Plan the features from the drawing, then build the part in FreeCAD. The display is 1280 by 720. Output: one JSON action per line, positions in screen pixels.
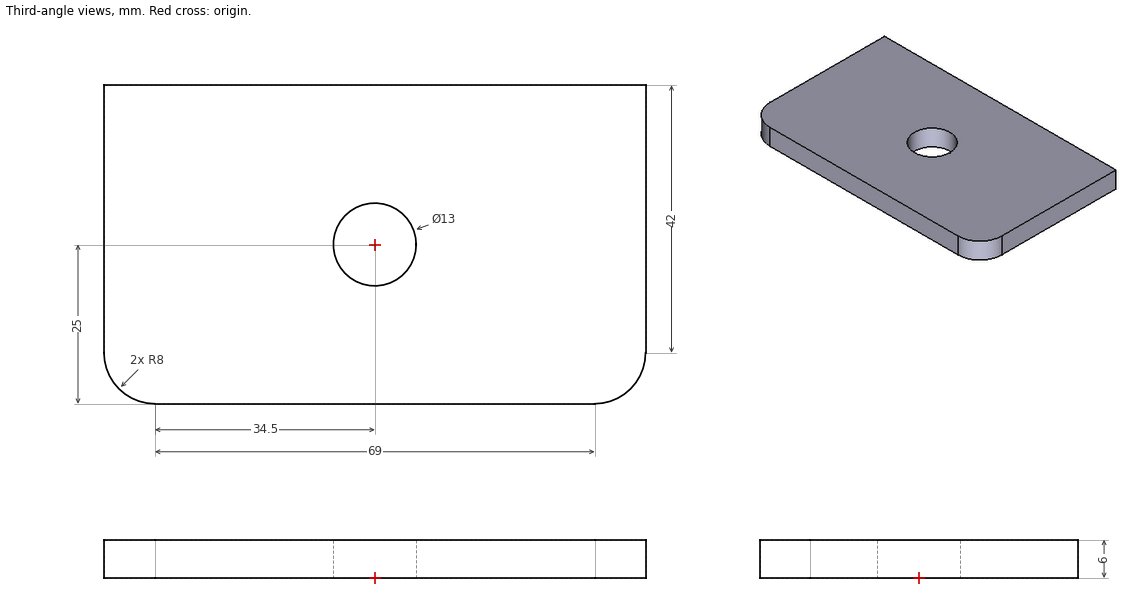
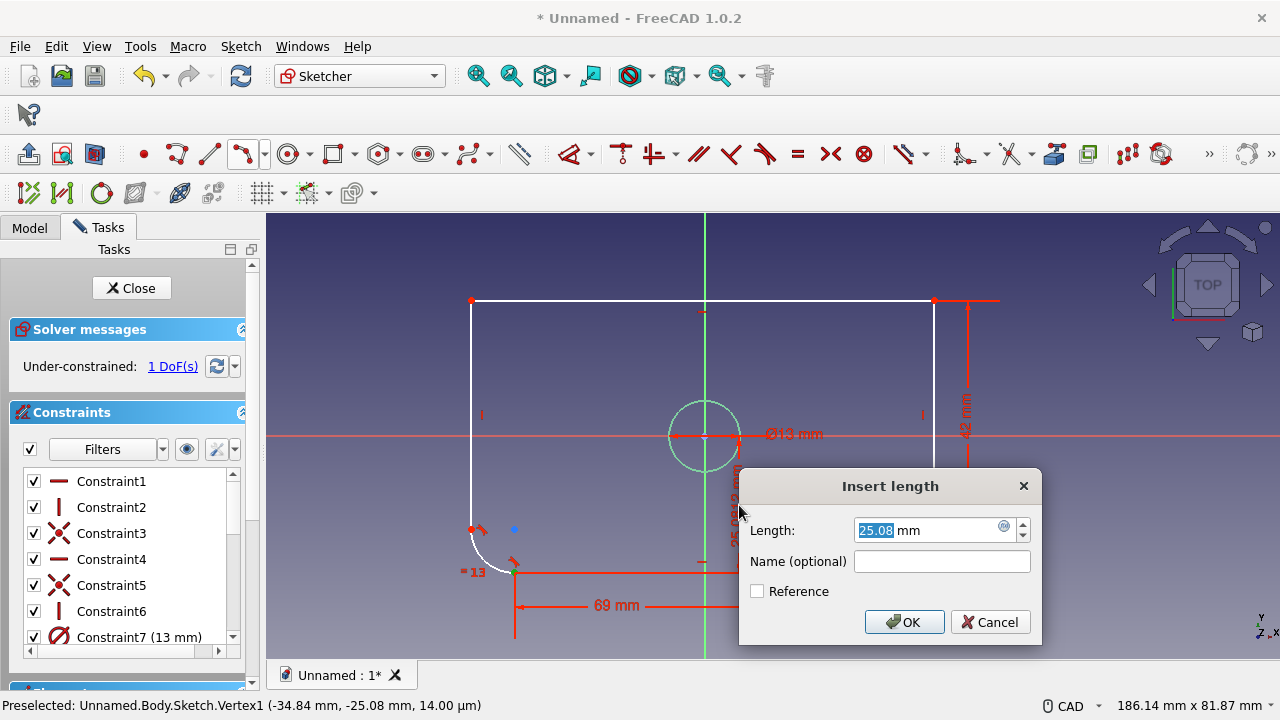
{"action": "type", "text": "25"}
{"action": "key", "text": "Return"}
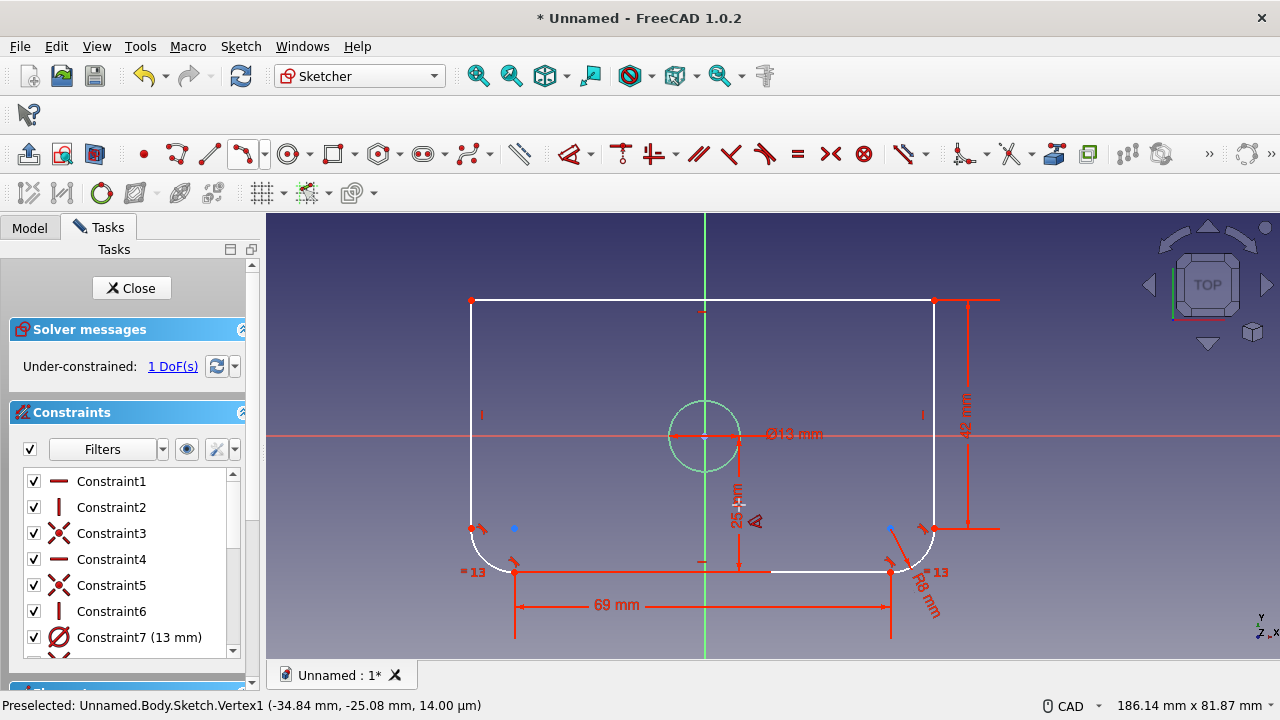
{"action": "left_click", "coordinate": [515, 572]}
{"action": "left_click", "coordinate": [543, 606]}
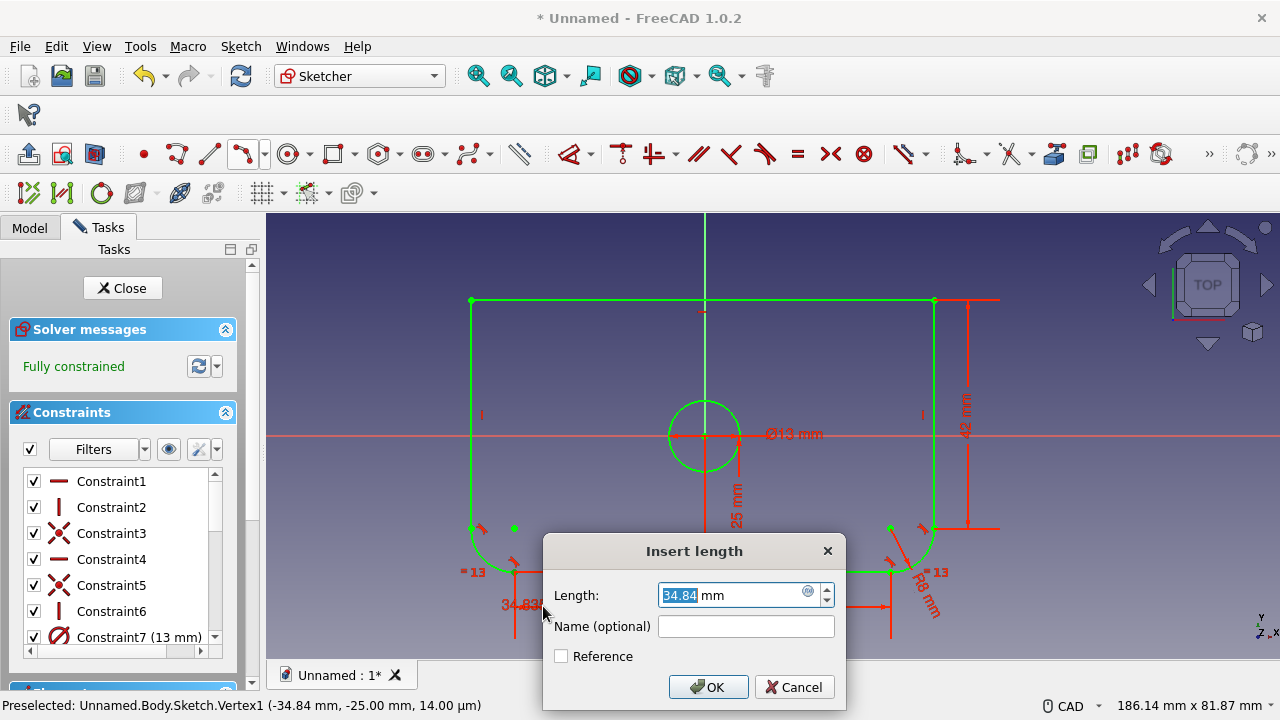
{"action": "type", "text": "34.5"}
{"action": "key", "text": "Return"}
{"action": "key", "text": "Escape"}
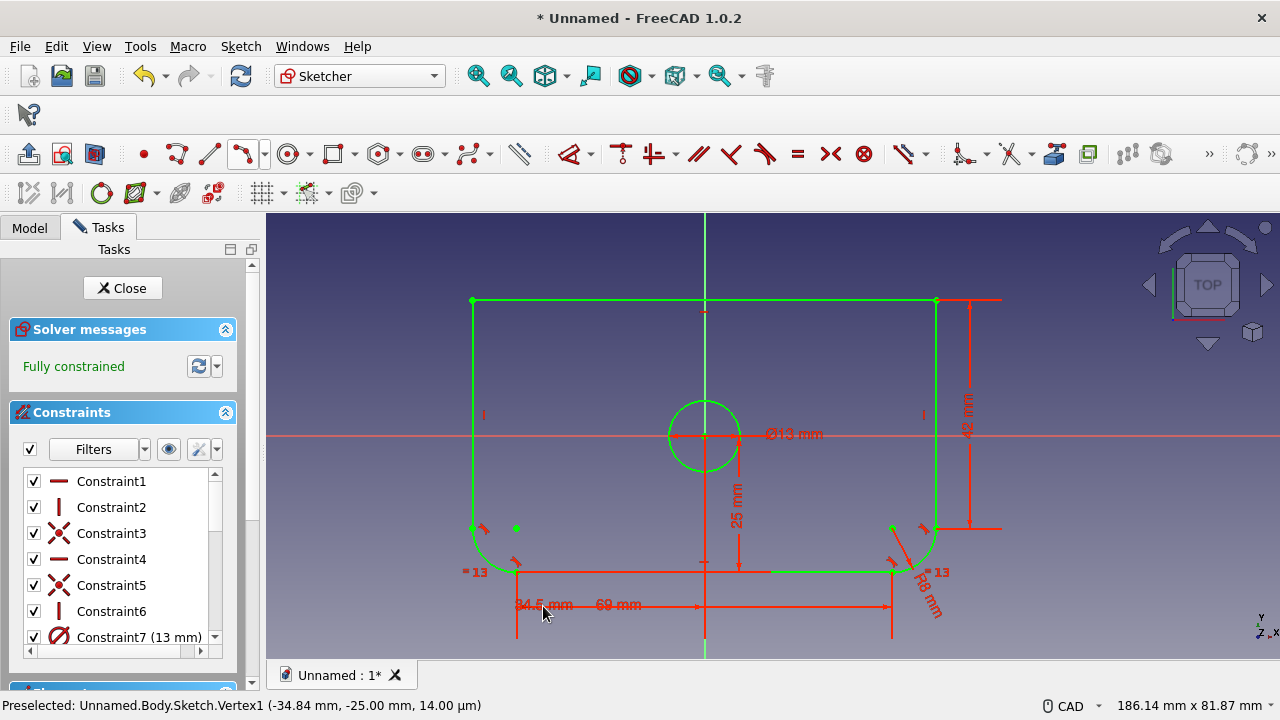
{"action": "left_click", "coordinate": [123, 288]}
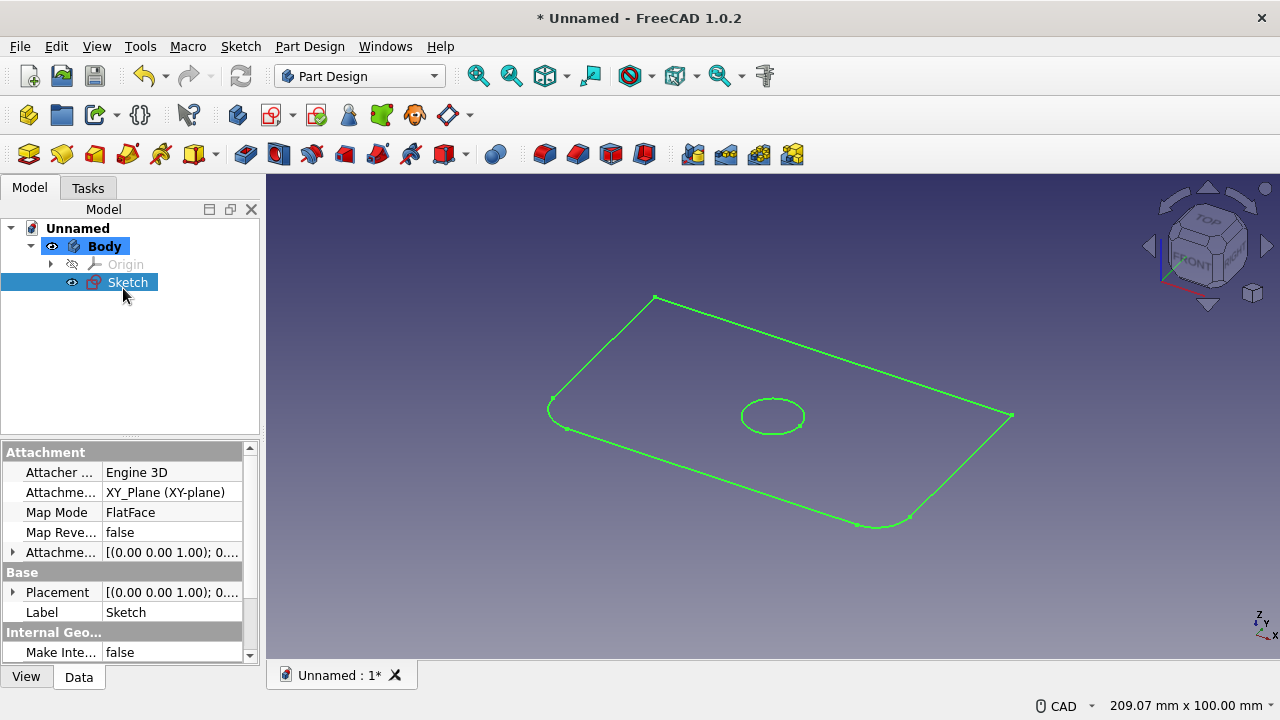
{"action": "left_click", "coordinate": [29, 154]}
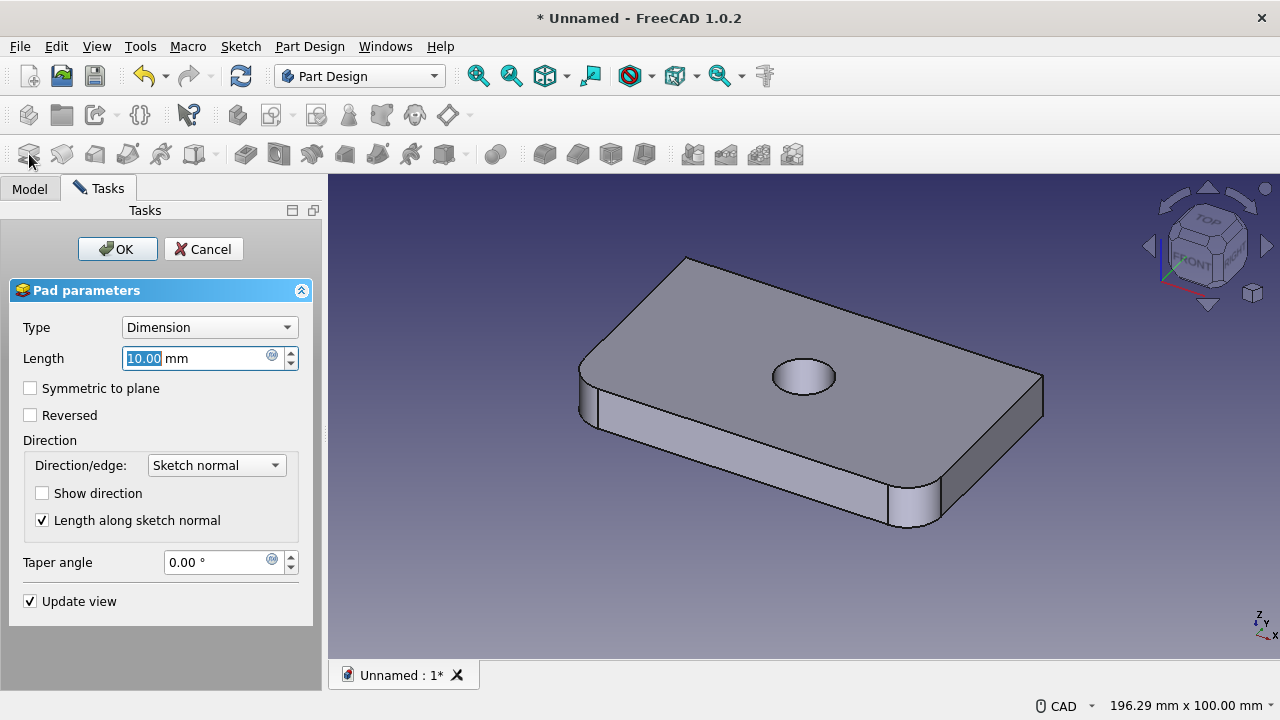
{"action": "type", "text": "6"}
{"action": "key", "text": "Tab"}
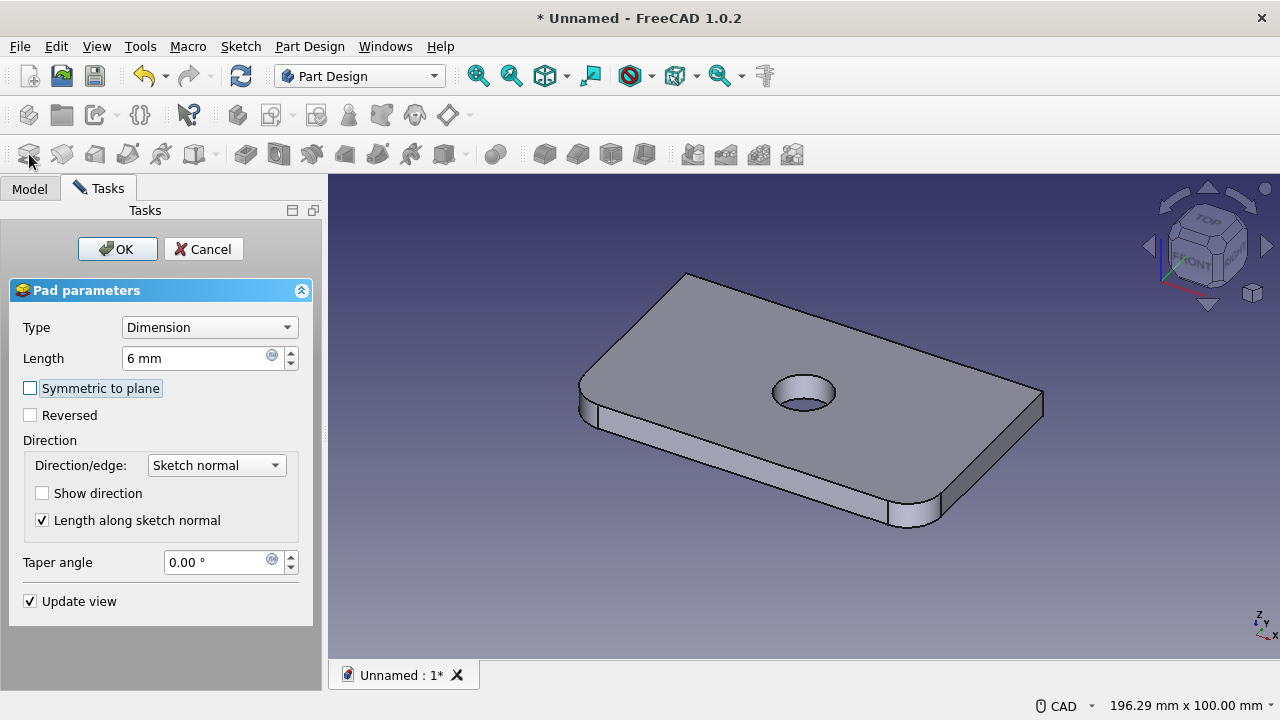
{"action": "left_click", "coordinate": [118, 249]}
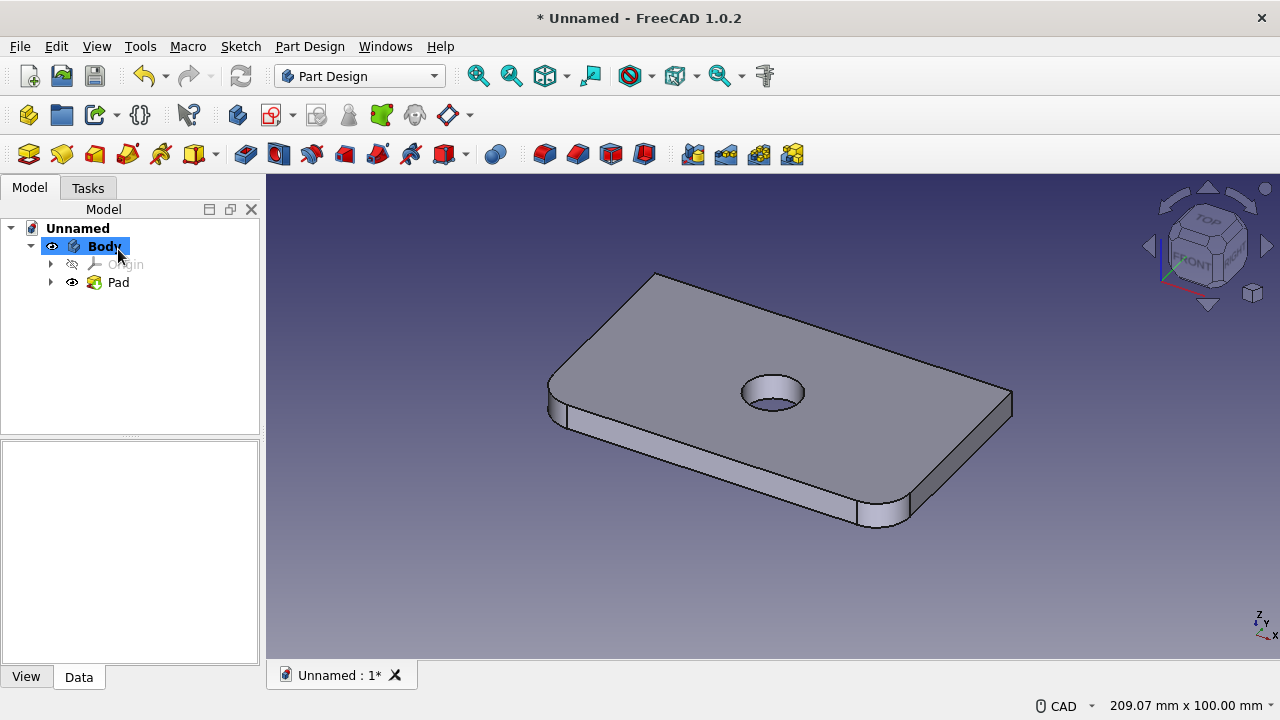
{"action": "key", "text": "0"}